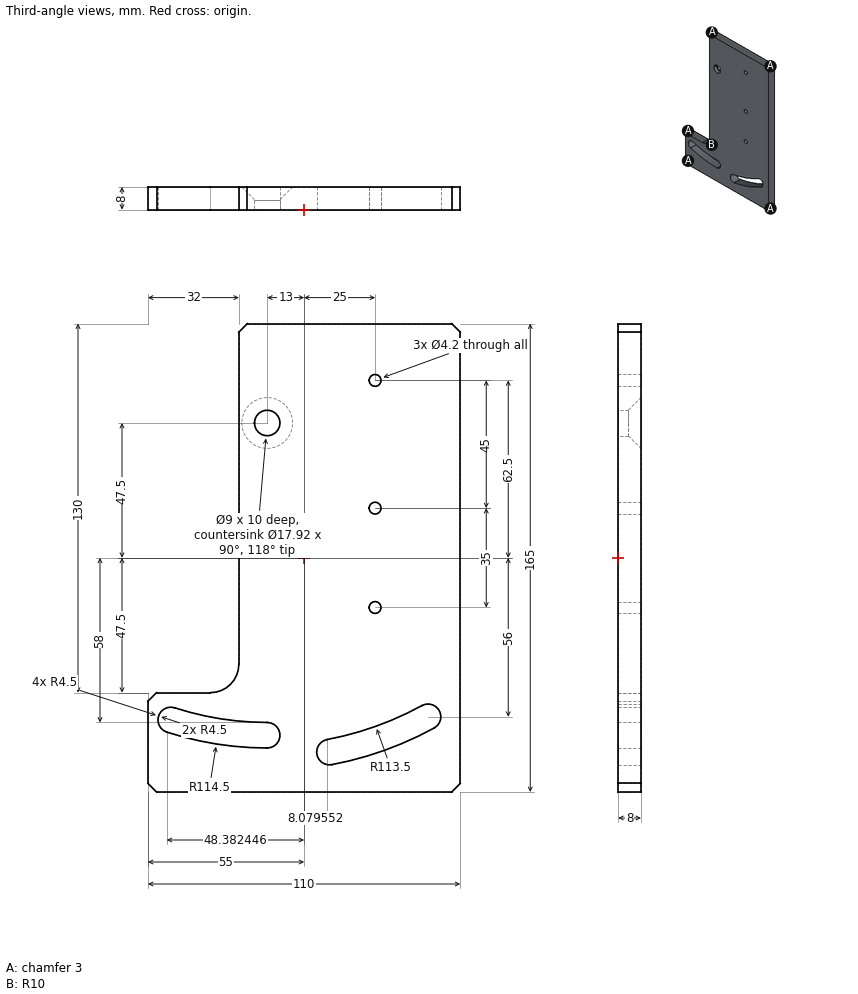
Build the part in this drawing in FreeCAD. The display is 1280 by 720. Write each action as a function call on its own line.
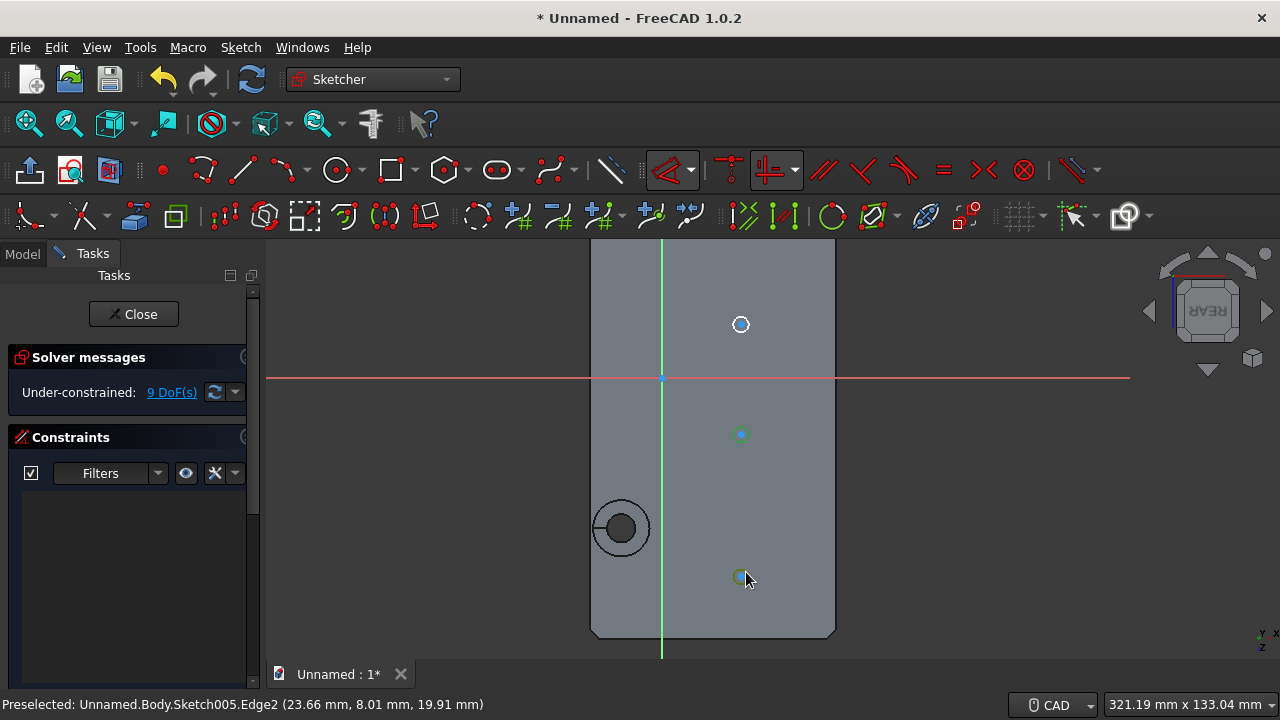
scroll(746, 319, up, 3)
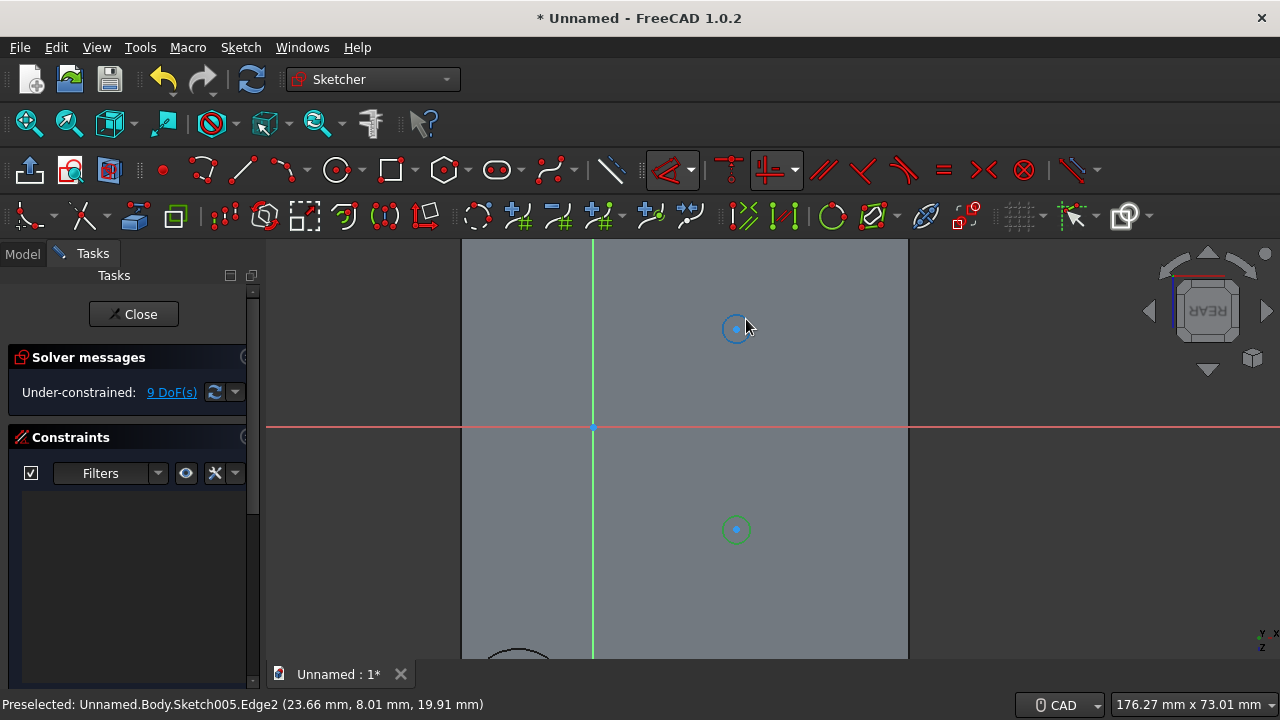
click(746, 319)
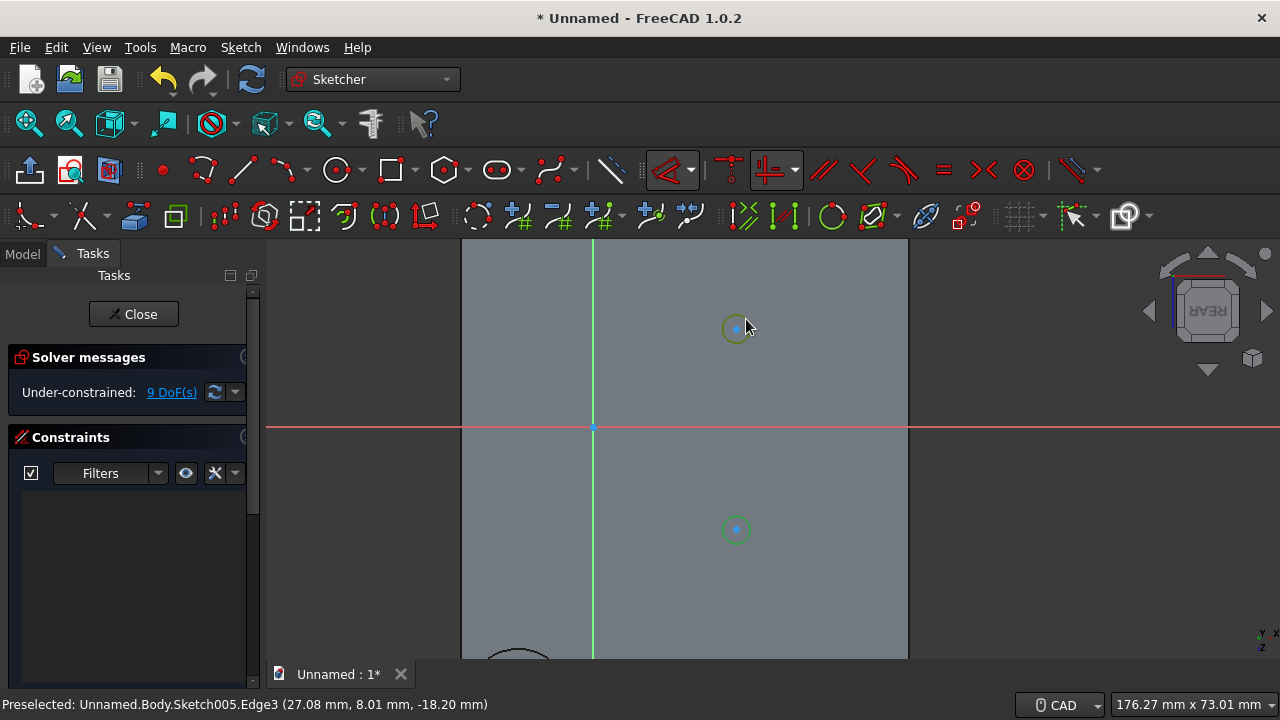
click(944, 170)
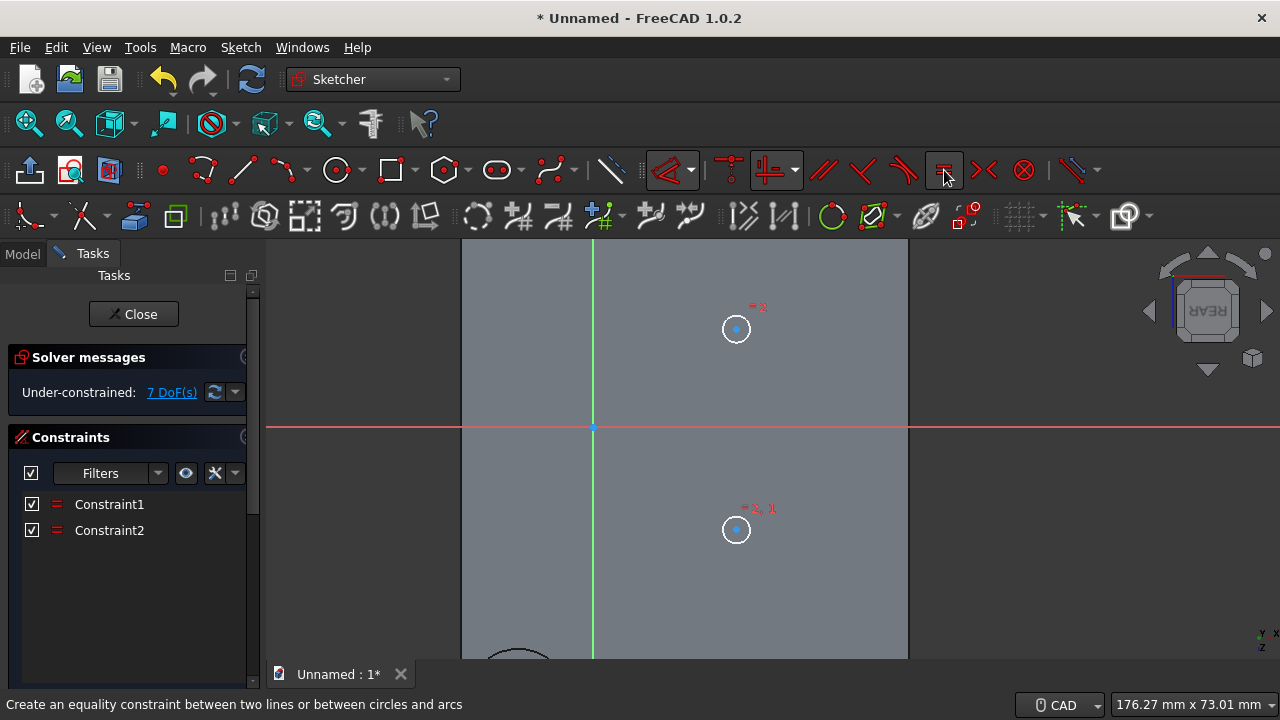
scroll(745, 318, down, 3)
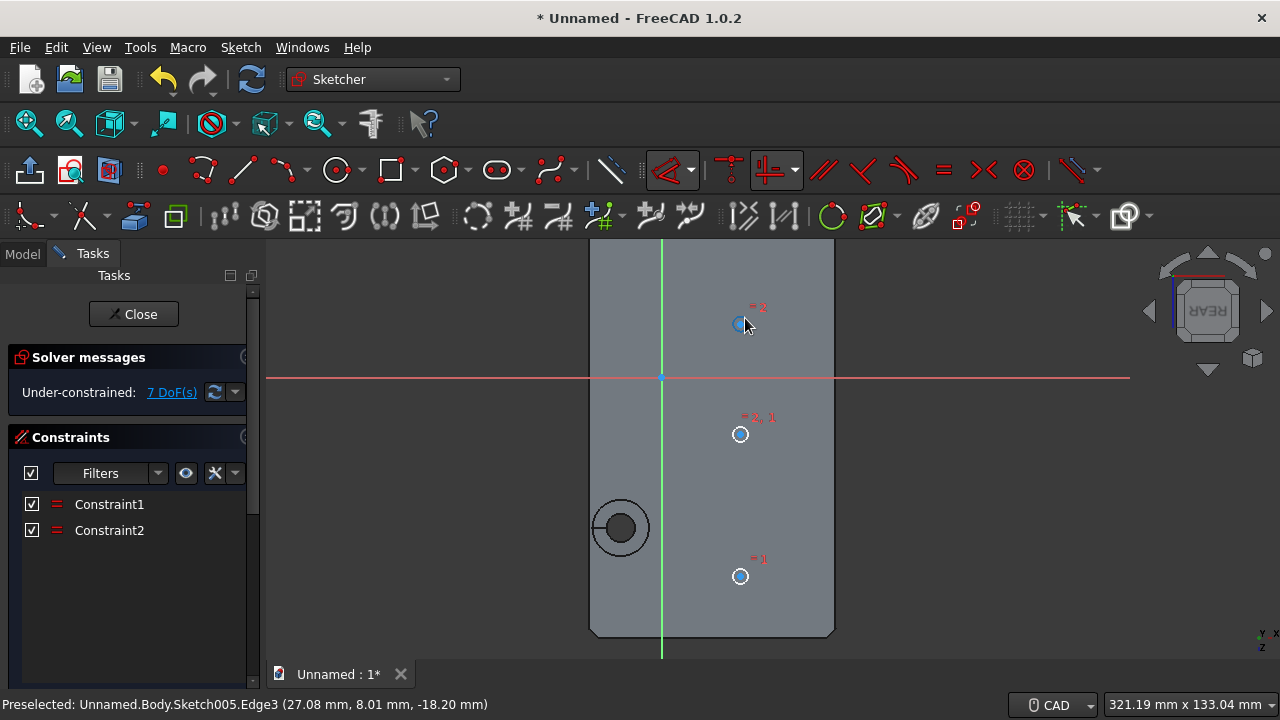
click(741, 576)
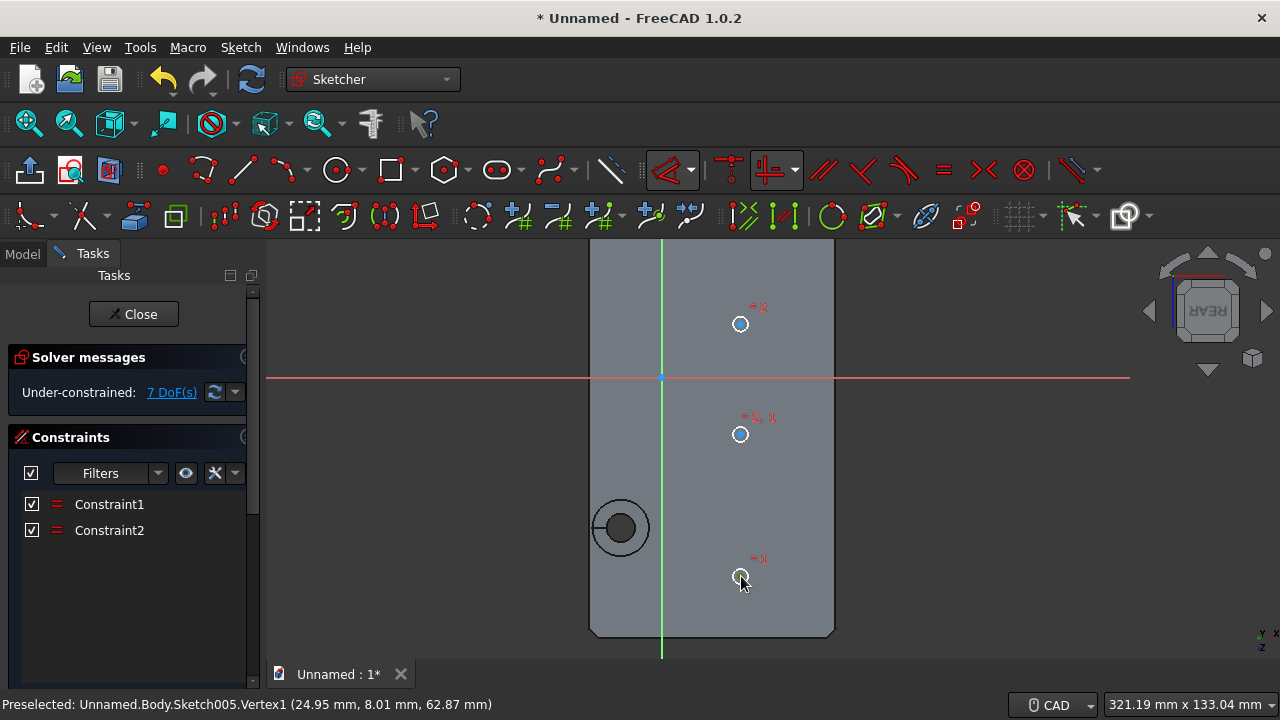
click(741, 434)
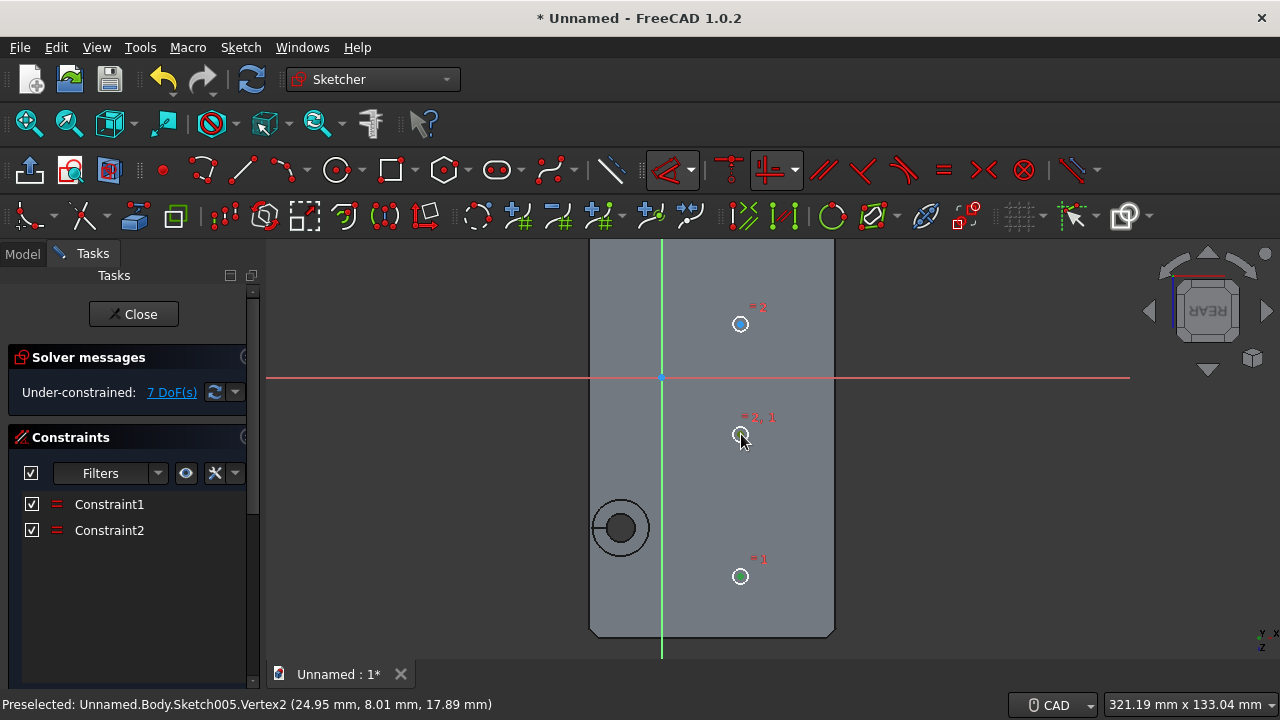
key(v)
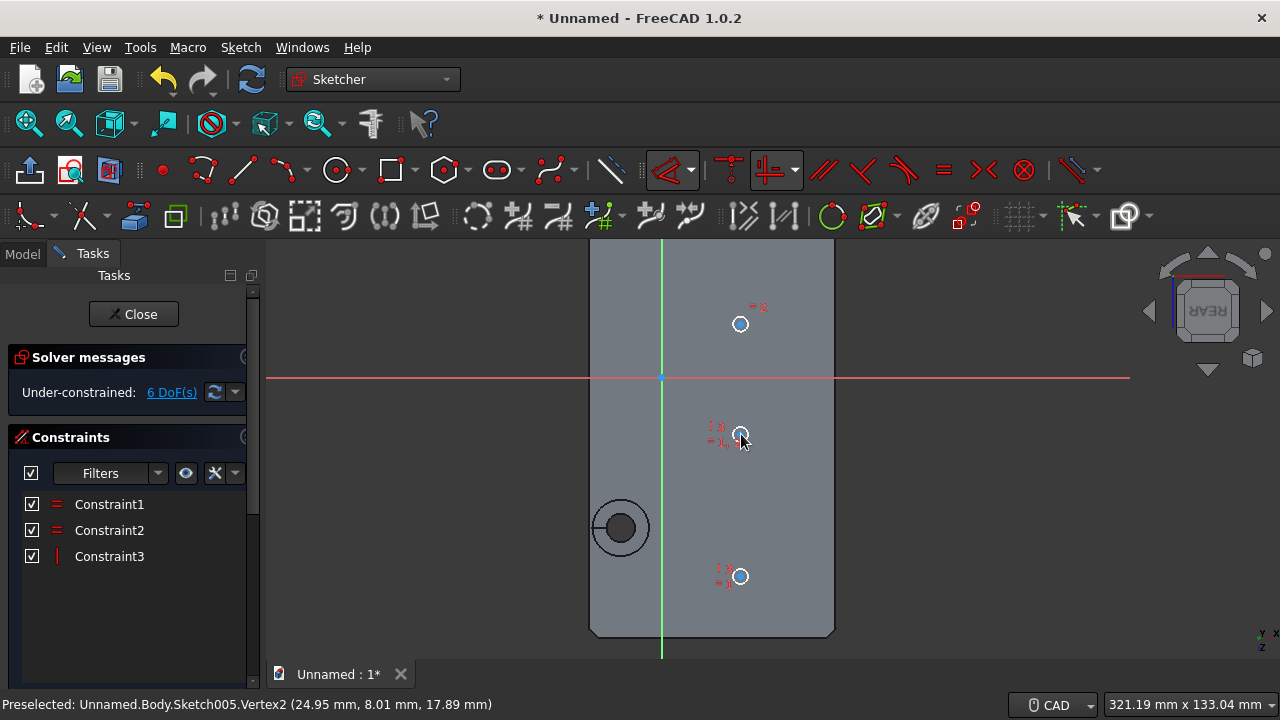
click(743, 436)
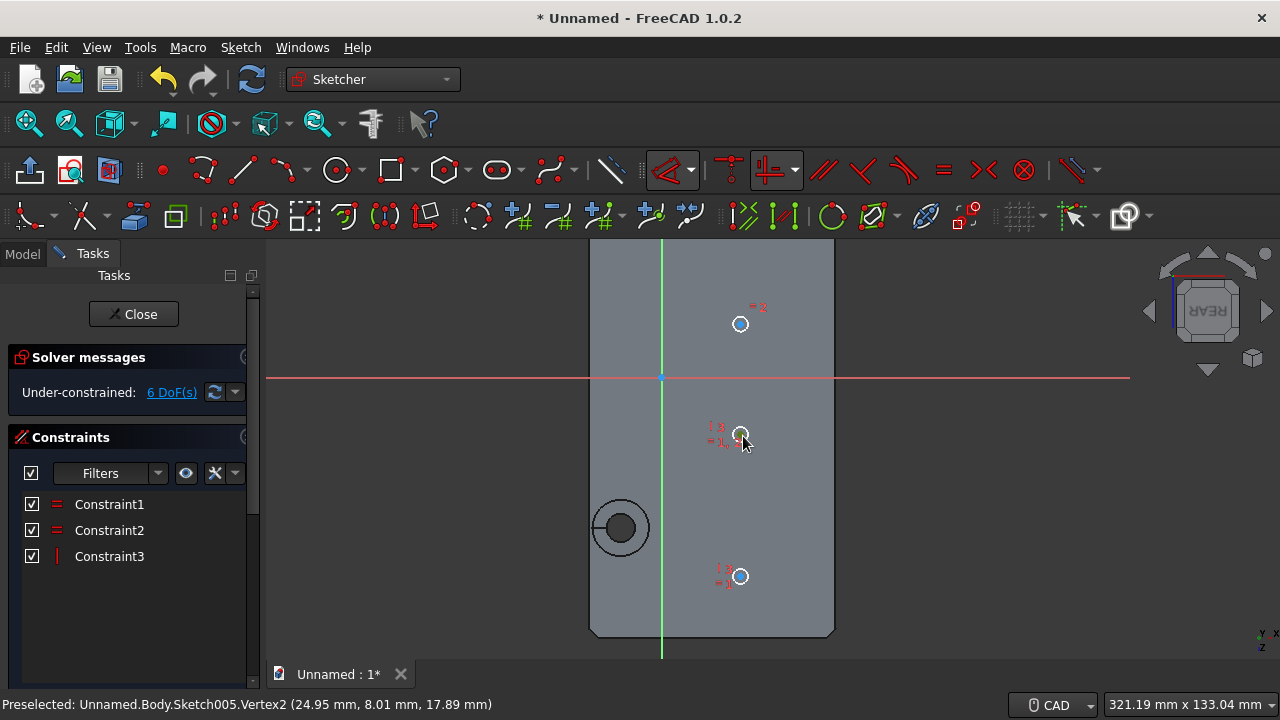
click(741, 324)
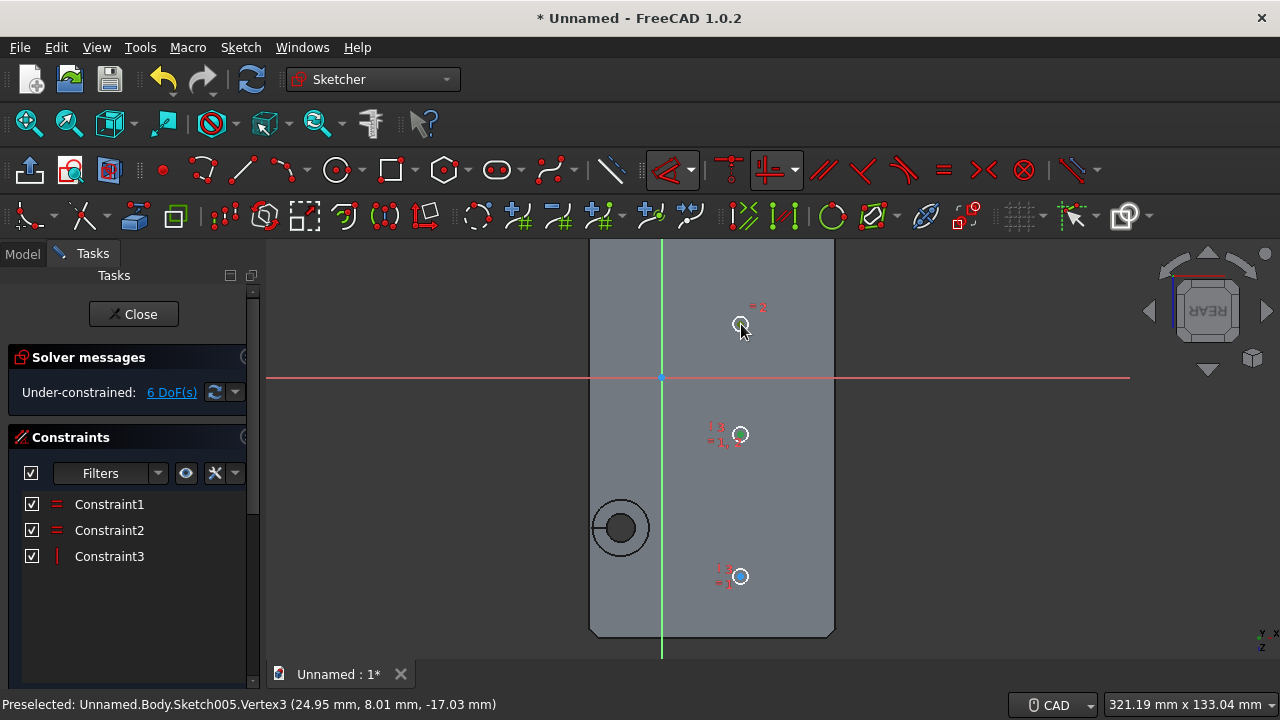
key(v)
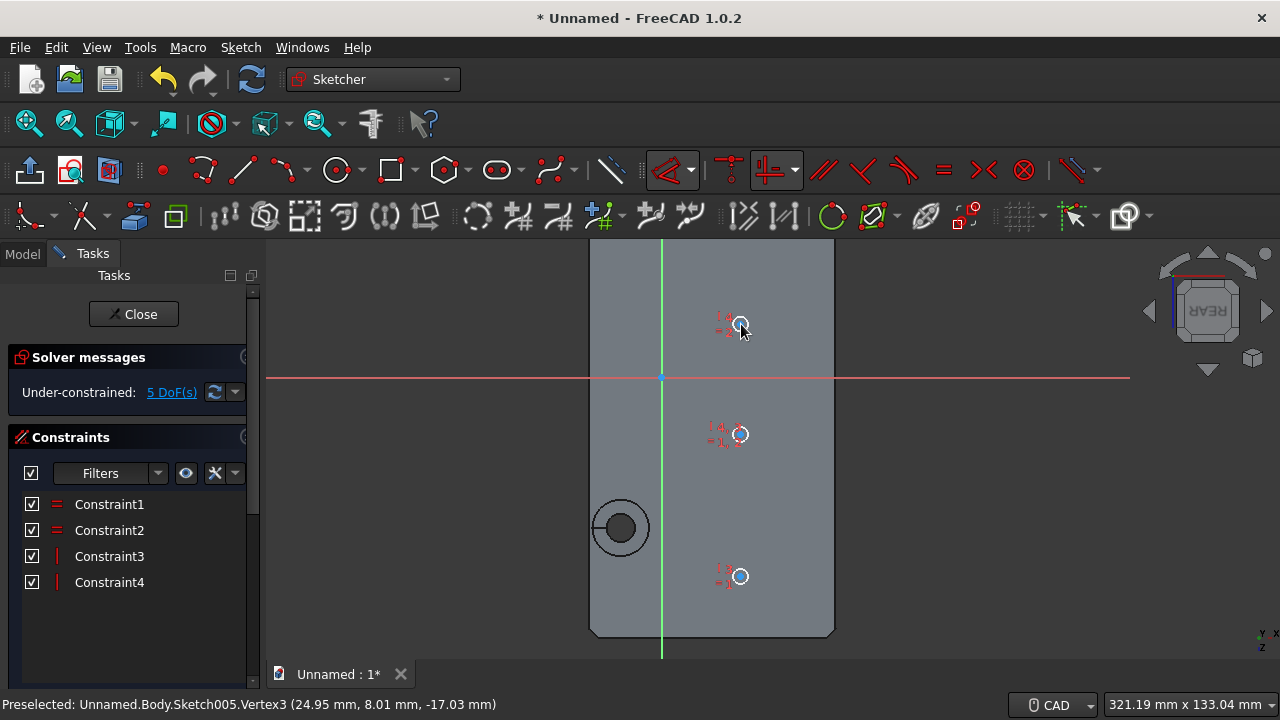
scroll(746, 571, up, 6)